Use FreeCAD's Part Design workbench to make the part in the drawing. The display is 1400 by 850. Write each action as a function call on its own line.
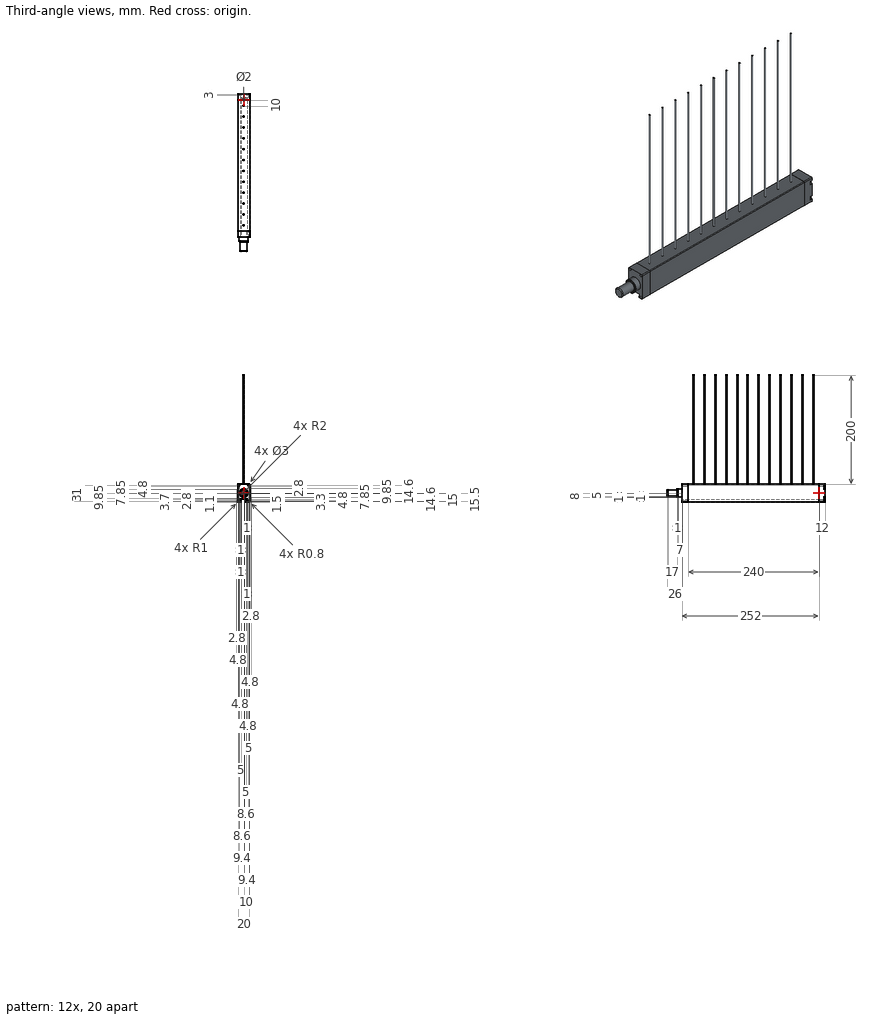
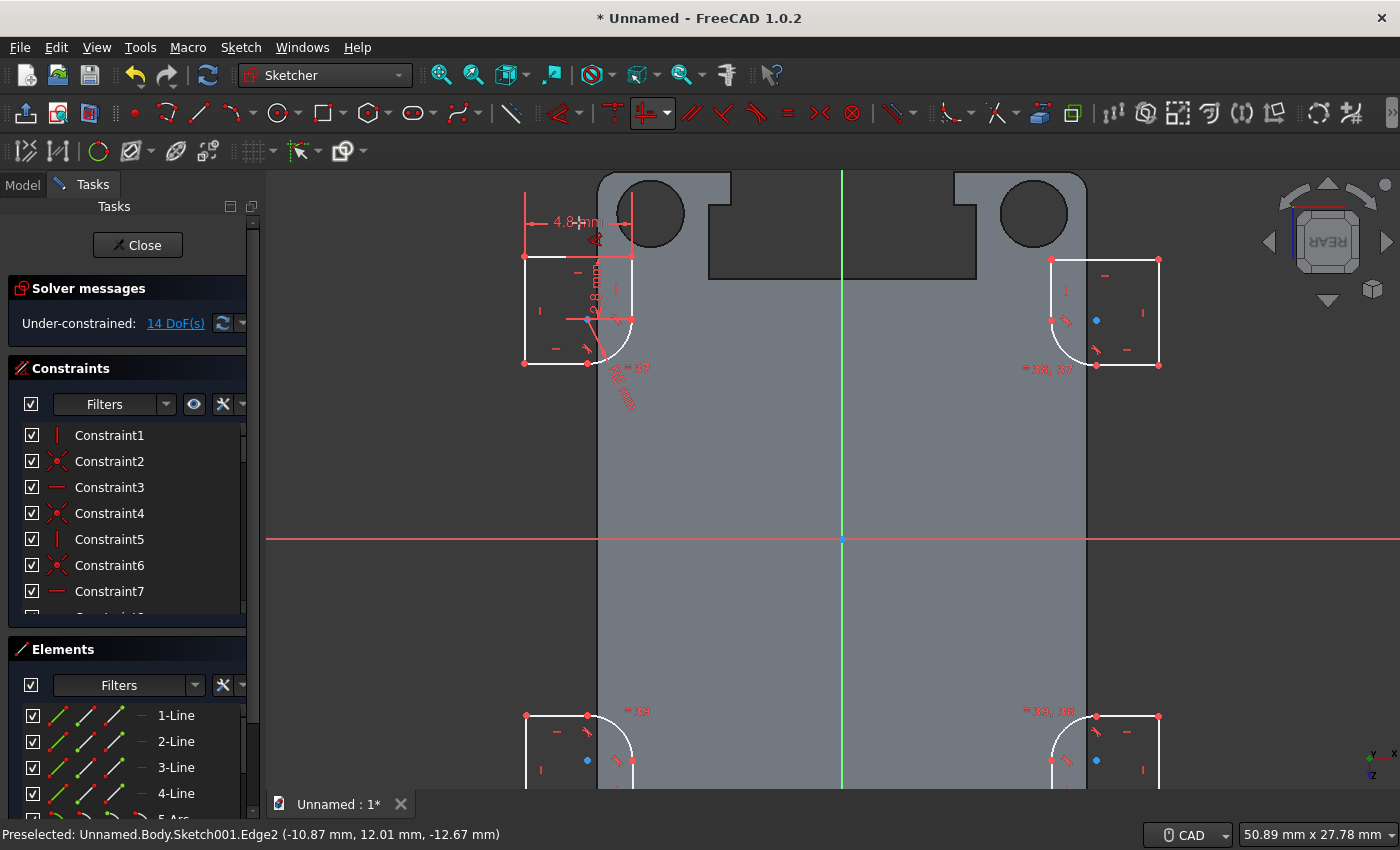
click(1115, 365)
click(1127, 331)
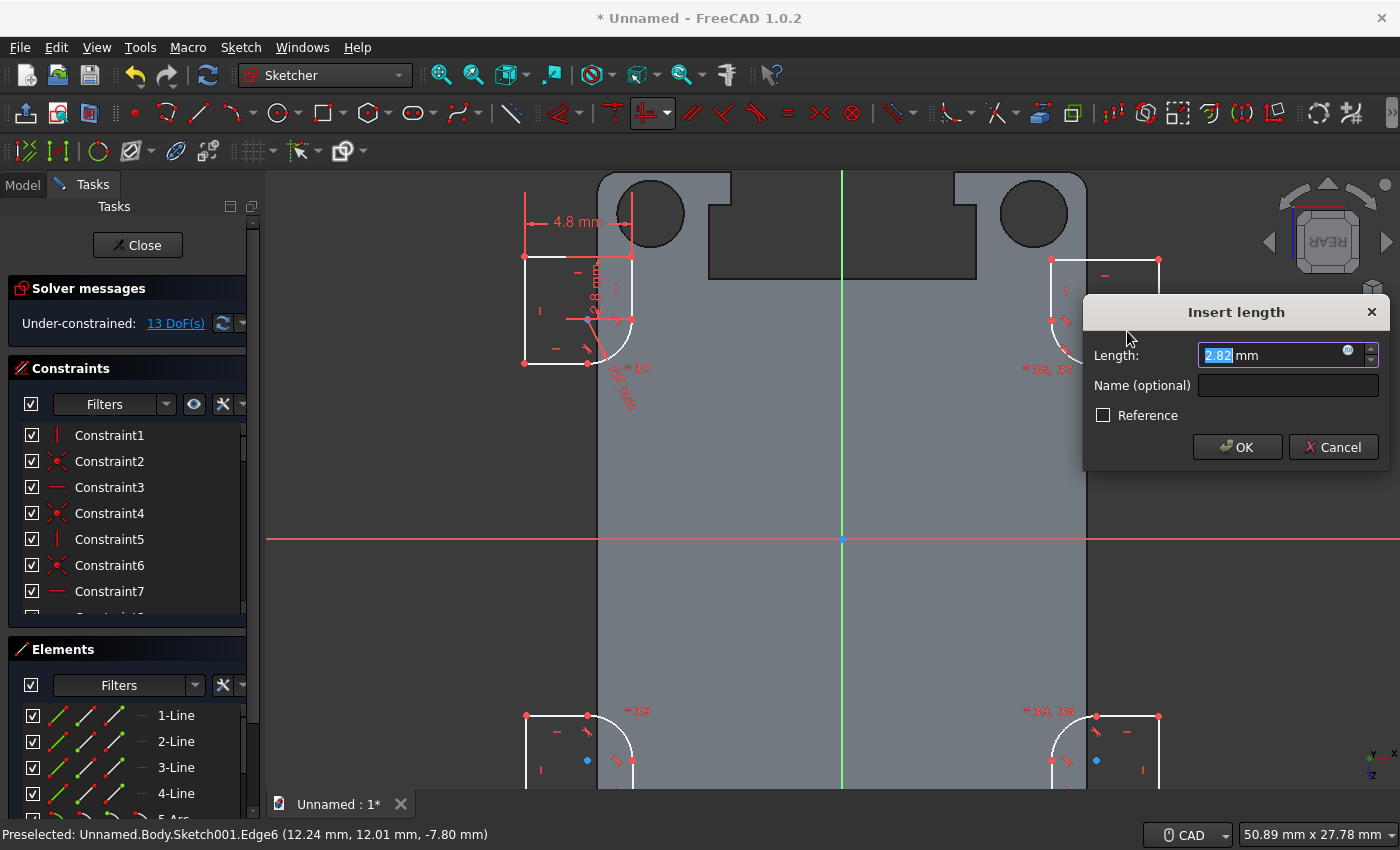
text(2.8)
key(Return)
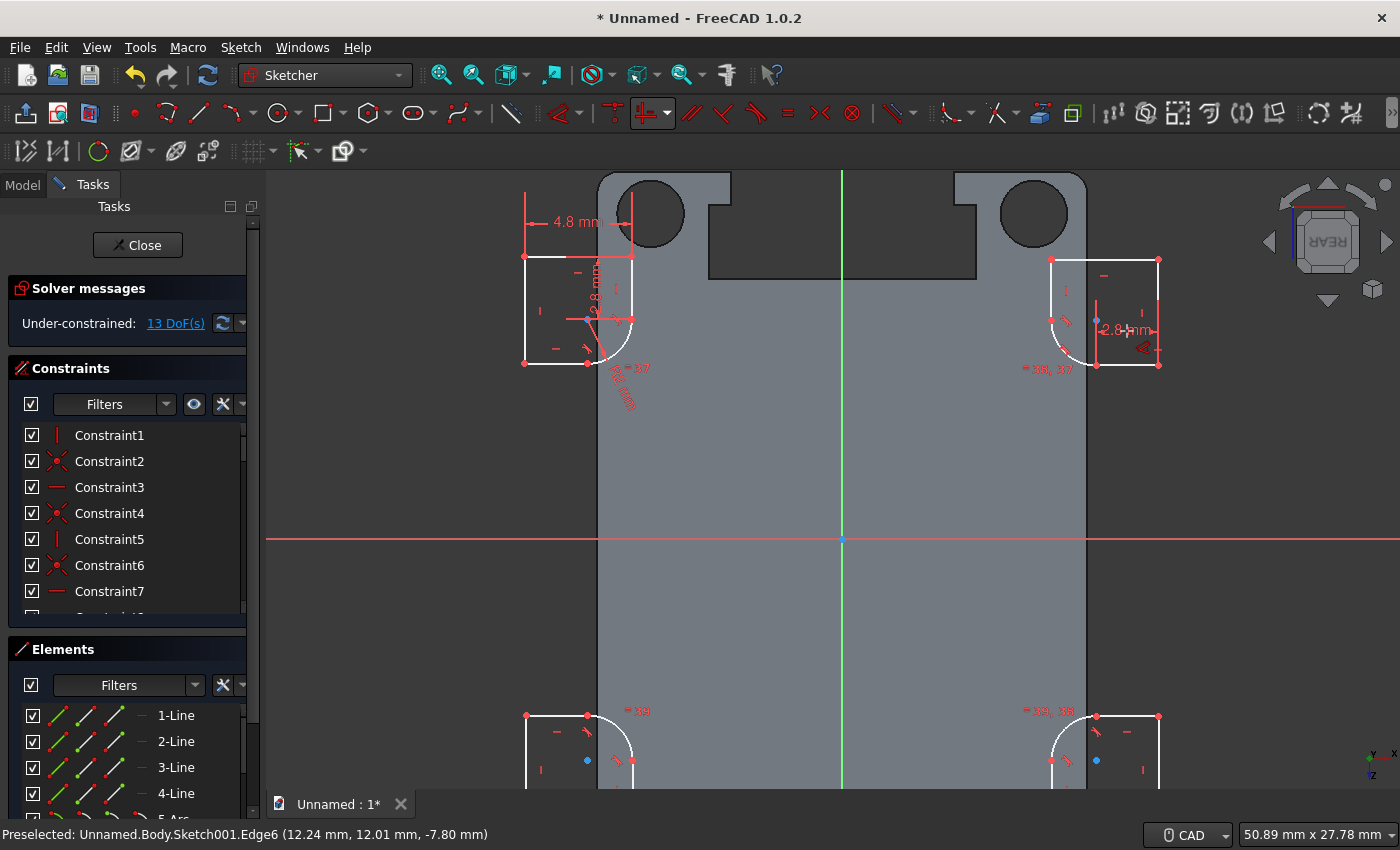
click(1158, 334)
click(1192, 288)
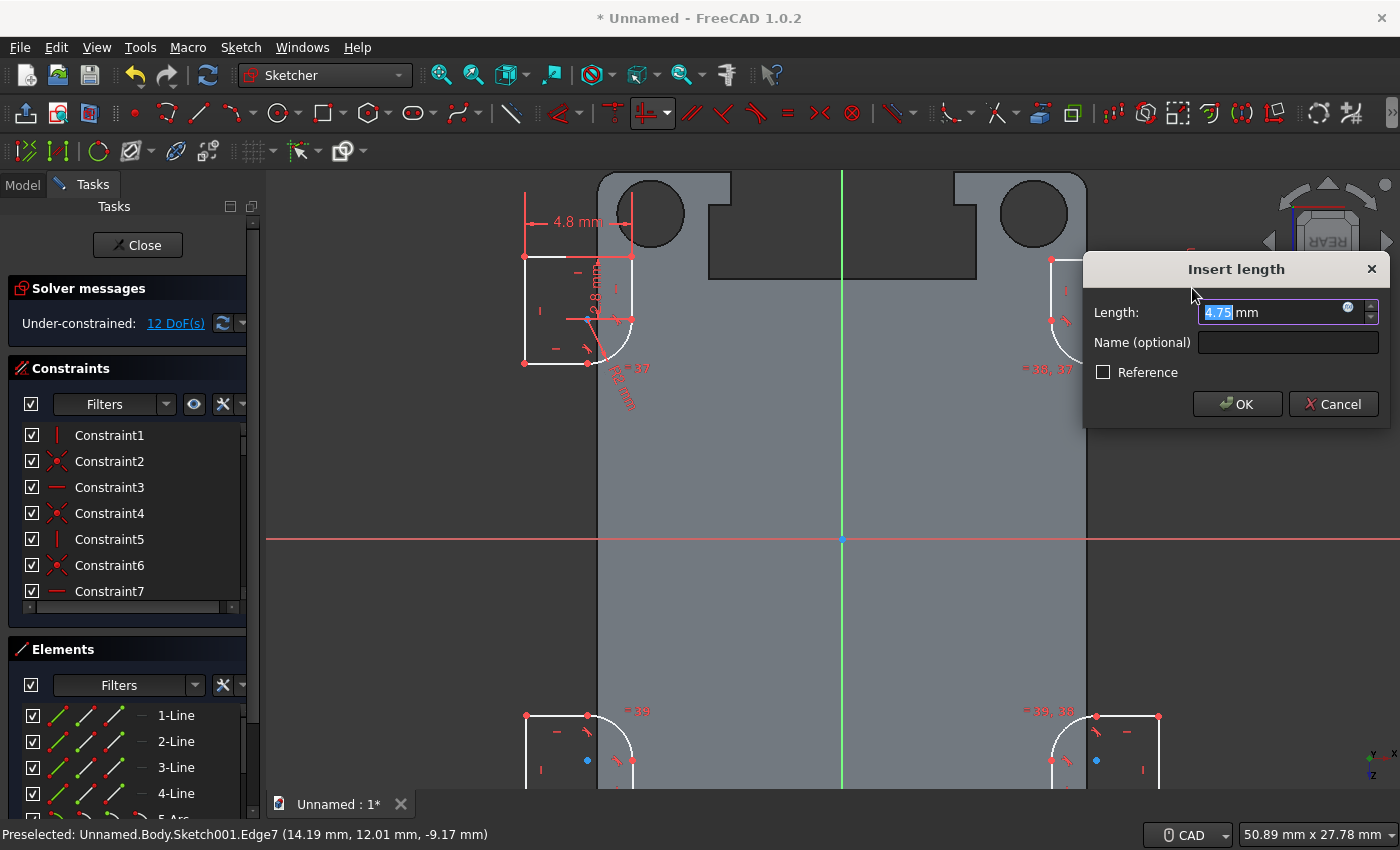
text(4.8)
key(Return)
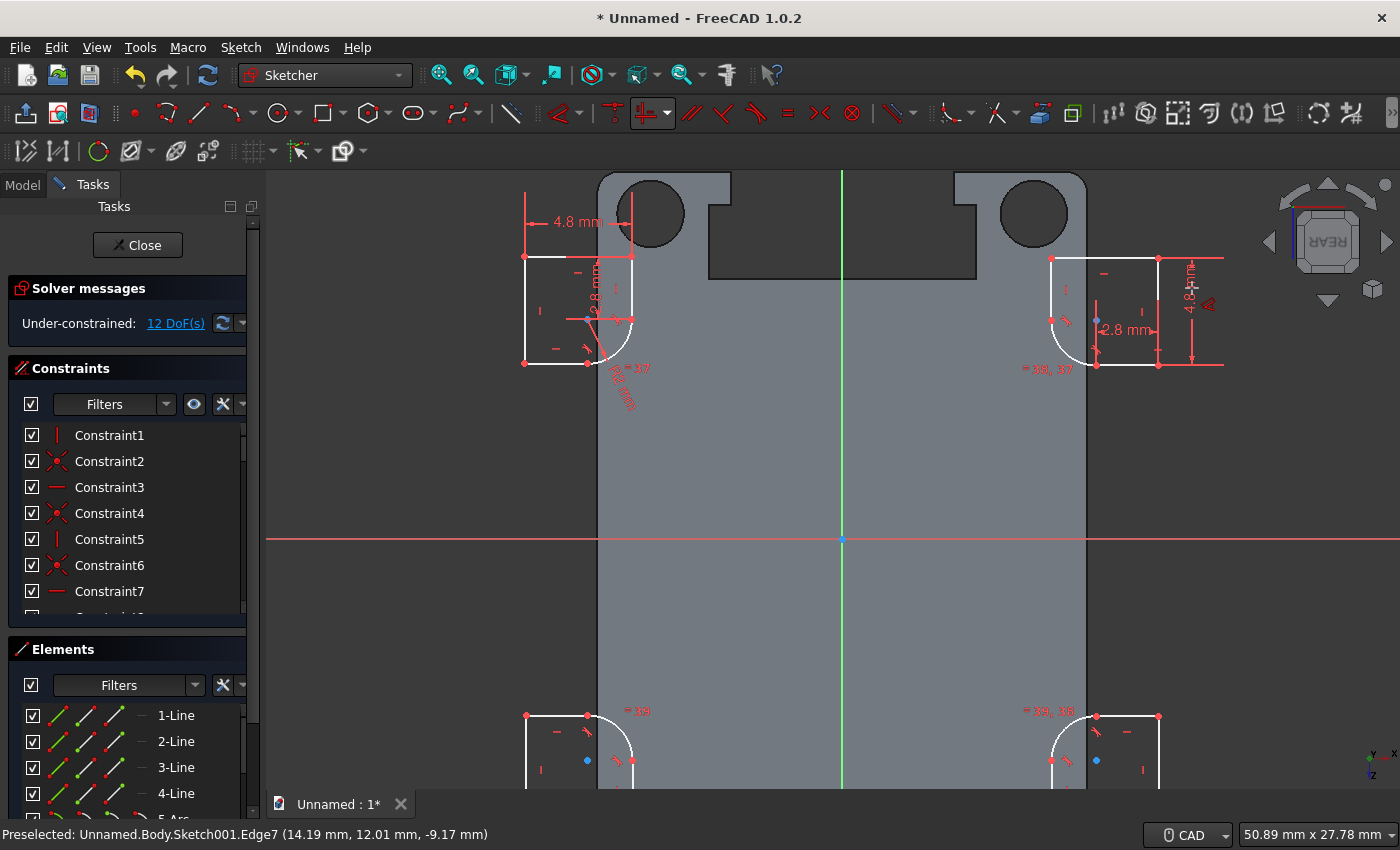
scroll(606, 358, down, 2)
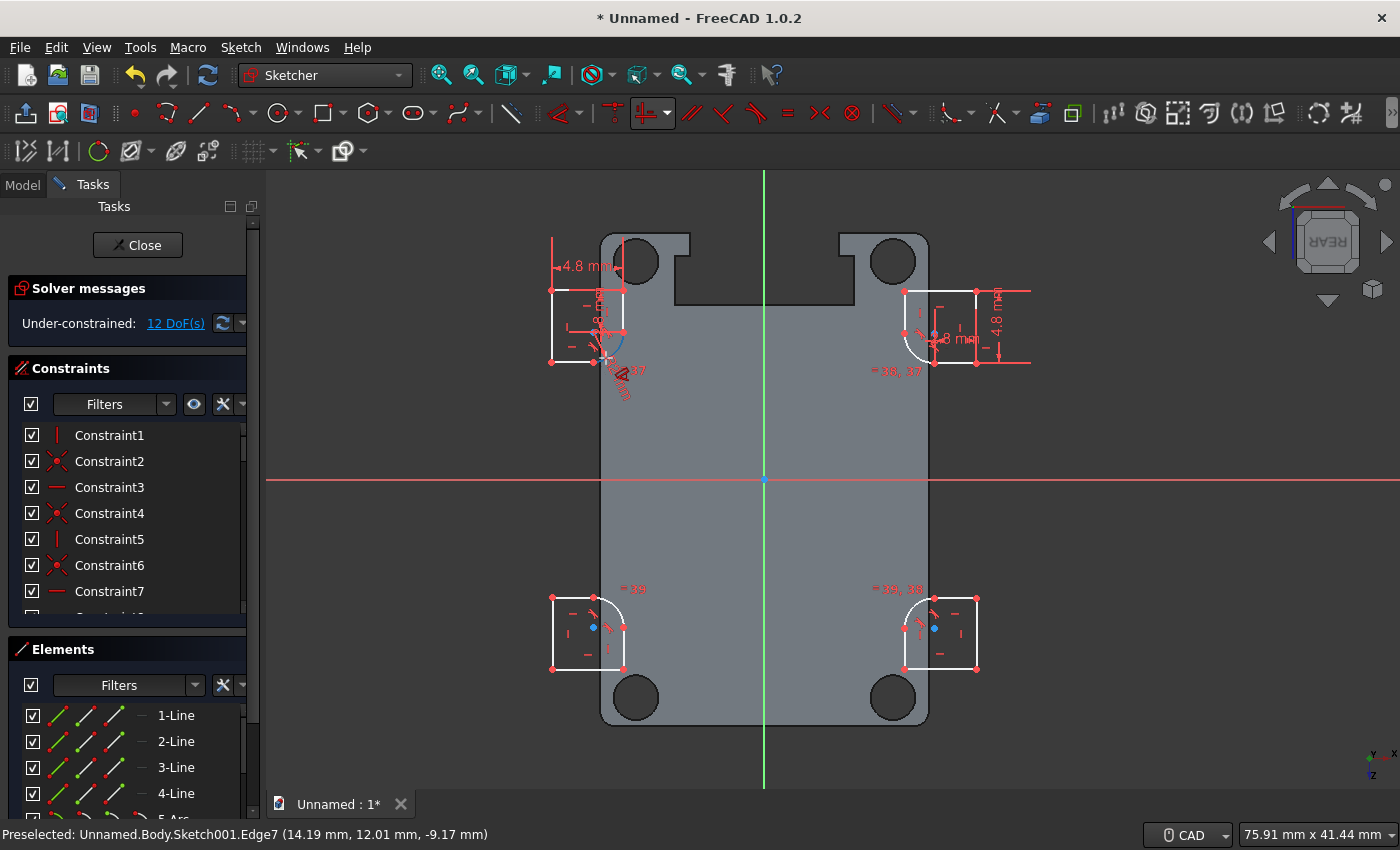
click(905, 640)
click(939, 649)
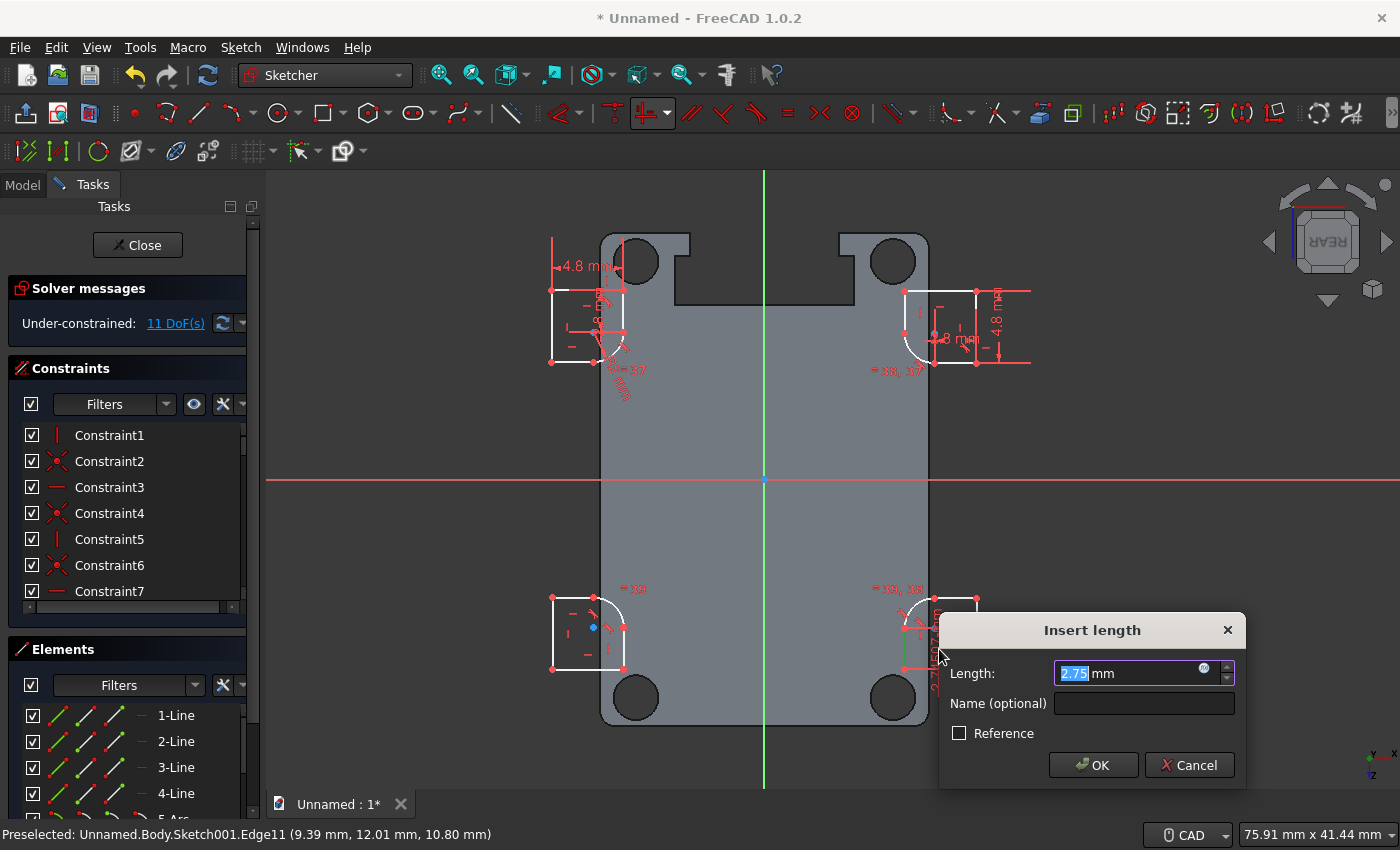
text(2.8)
key(Return)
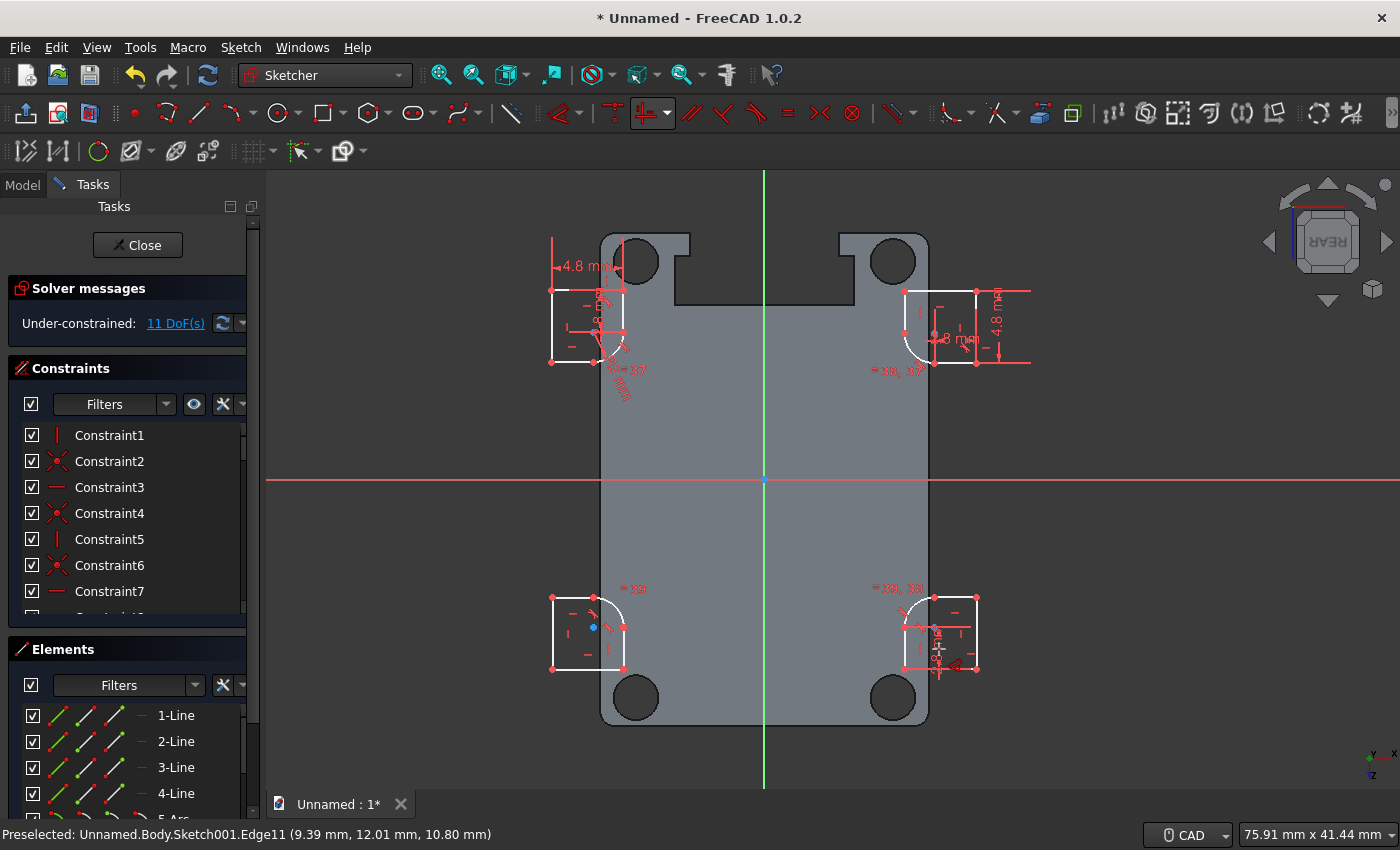
click(926, 669)
click(941, 703)